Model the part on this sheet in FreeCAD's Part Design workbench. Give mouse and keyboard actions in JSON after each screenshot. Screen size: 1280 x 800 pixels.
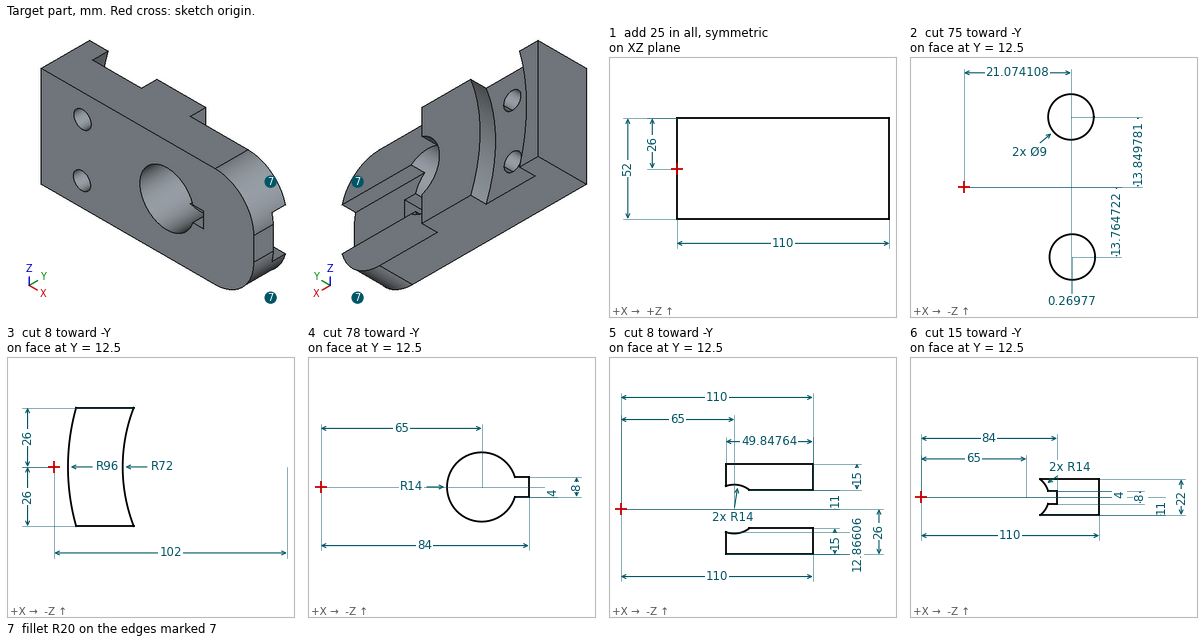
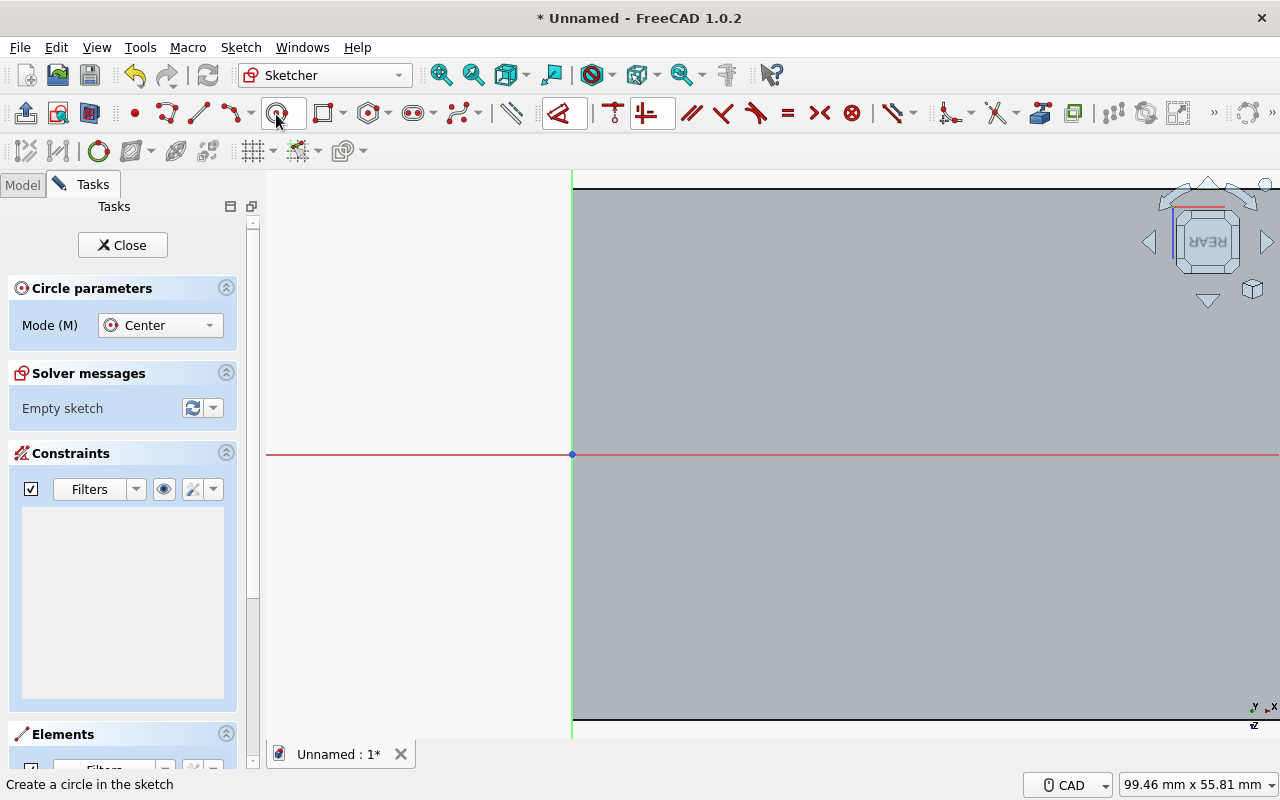
{"action": "left_click", "coordinate": [787, 313]}
{"action": "left_click", "coordinate": [820, 281]}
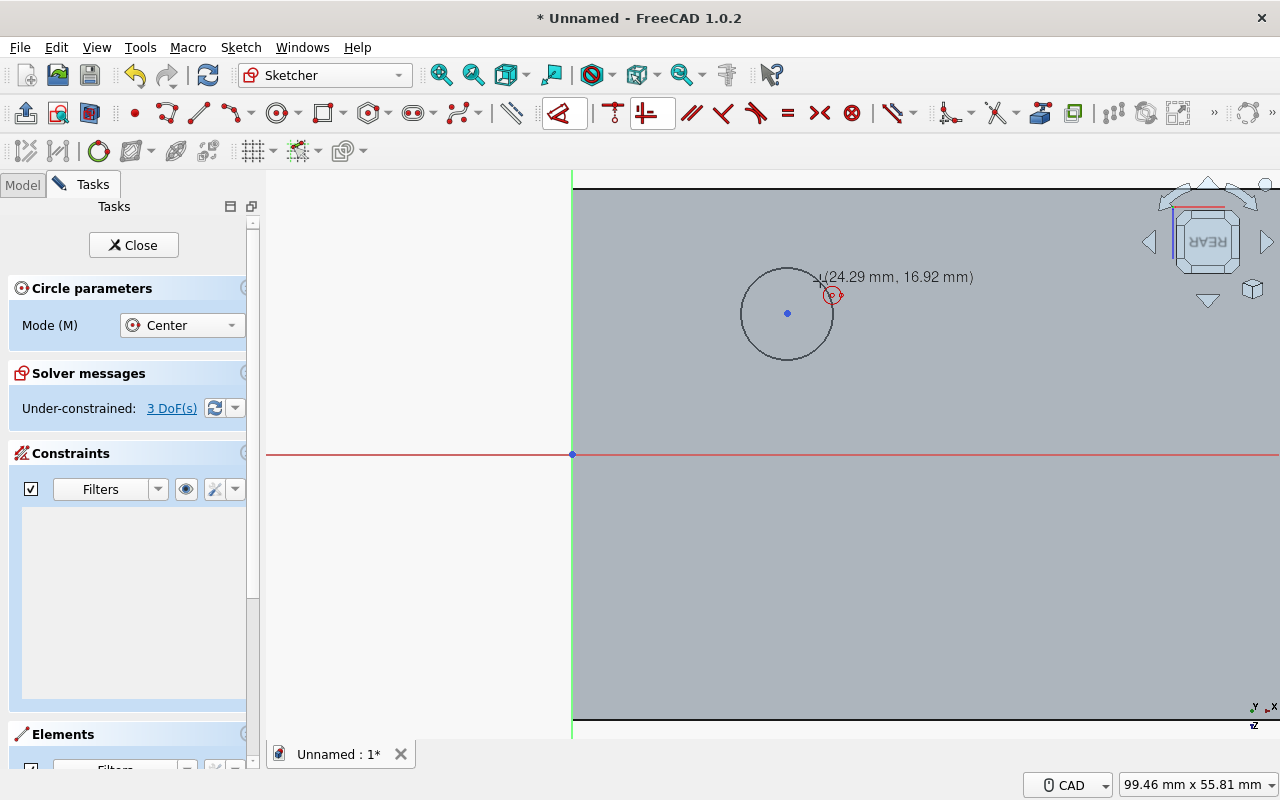
{"action": "left_click", "coordinate": [790, 595]}
{"action": "left_click", "coordinate": [822, 562]}
{"action": "key", "text": "Escape"}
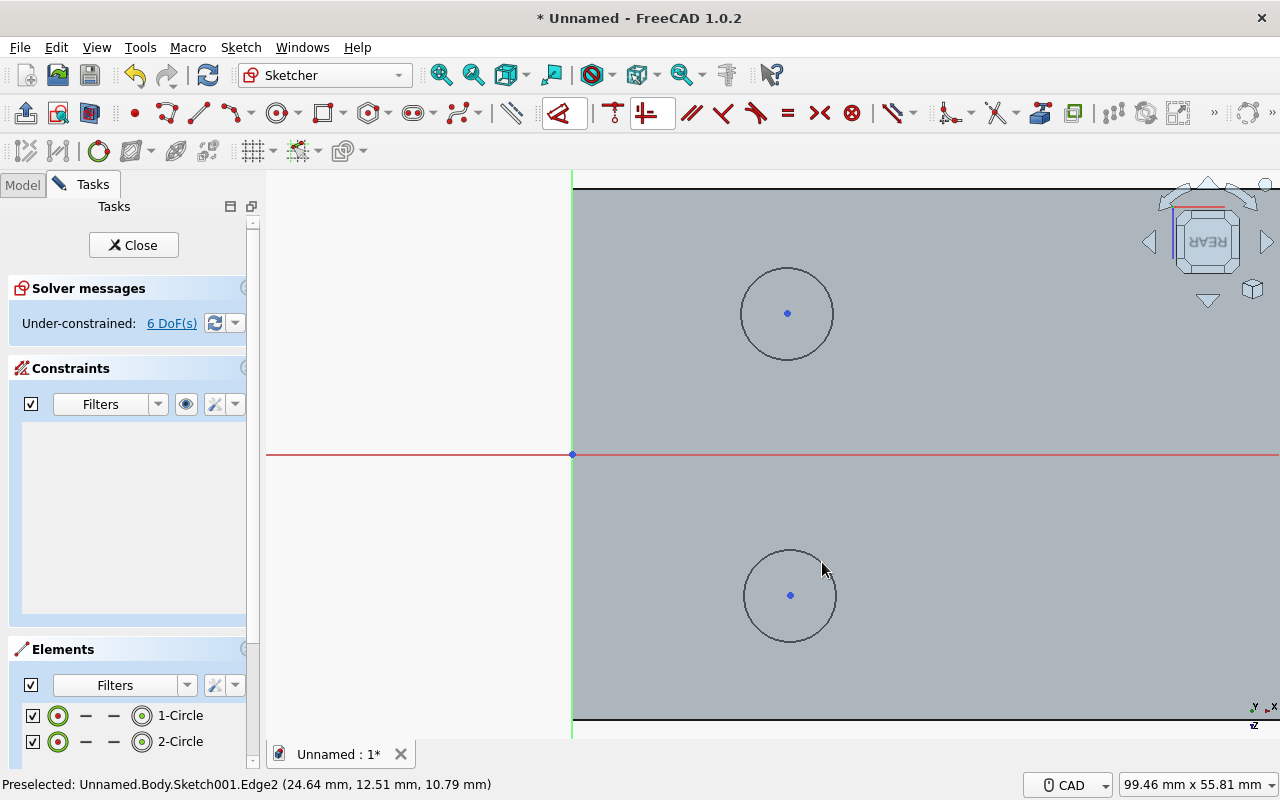
{"action": "left_click", "coordinate": [819, 281]}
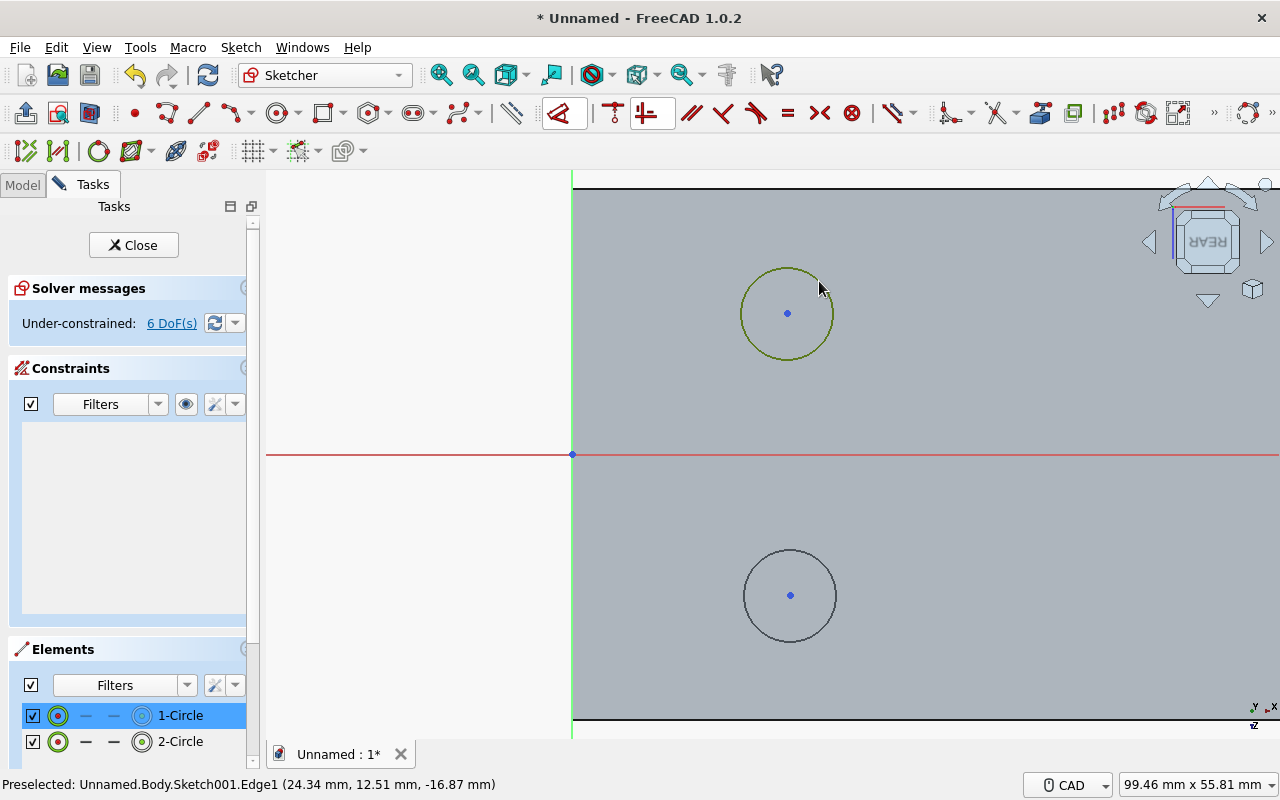
{"action": "left_click", "coordinate": [822, 563]}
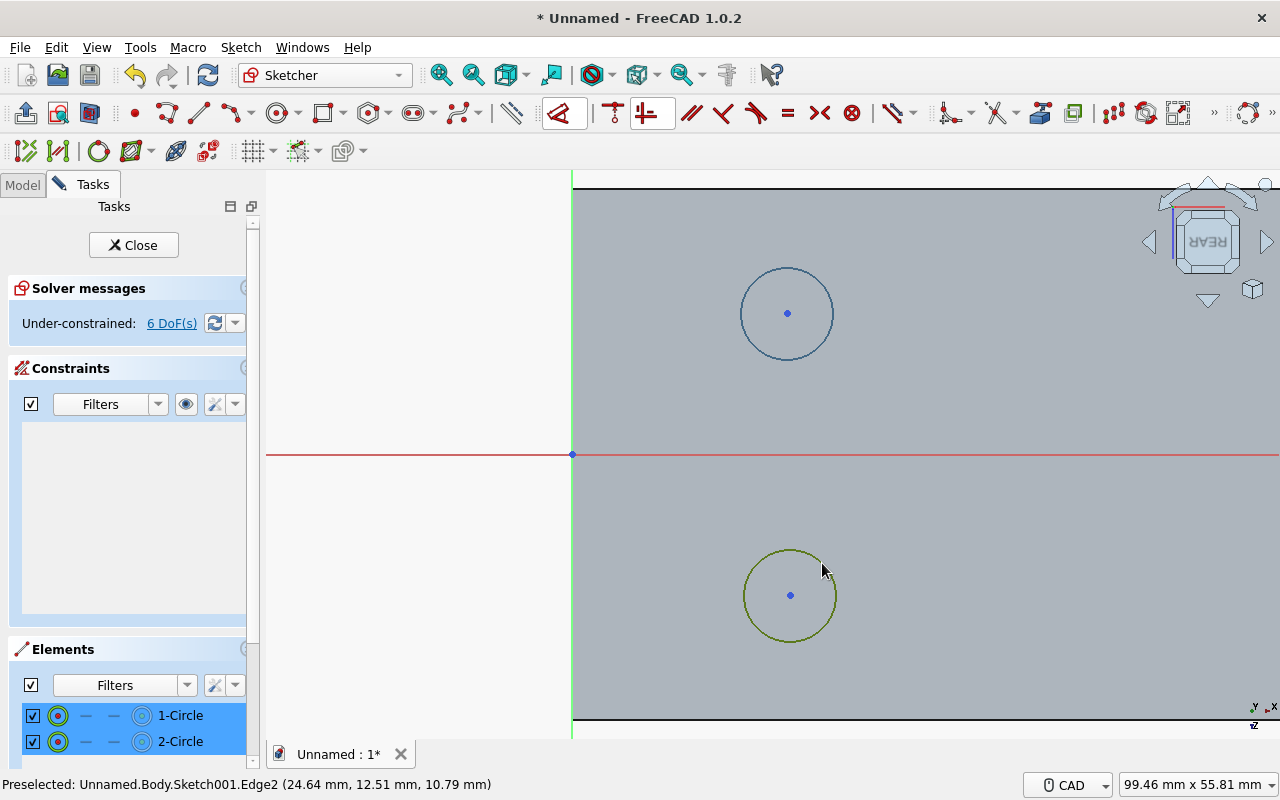
{"action": "left_click", "coordinate": [788, 114]}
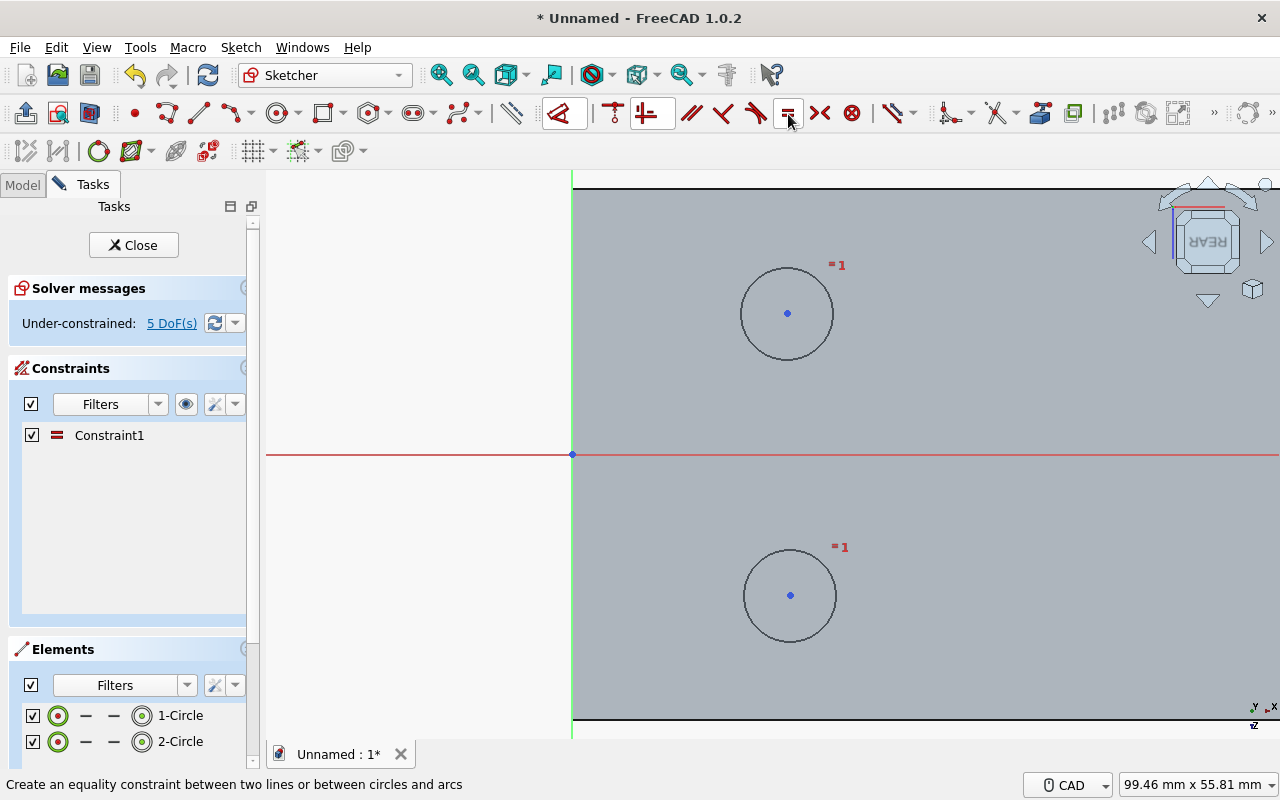
{"action": "left_click", "coordinate": [819, 281]}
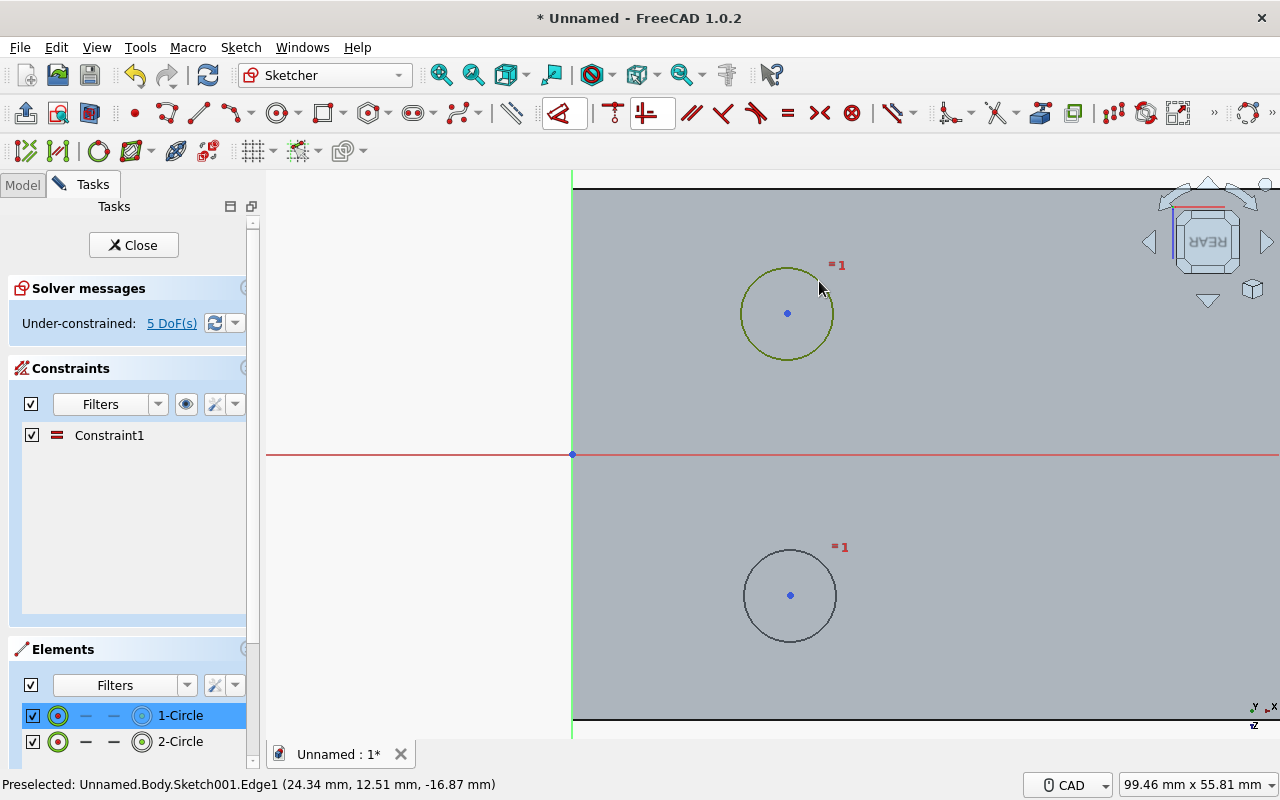
{"action": "left_click", "coordinate": [582, 114]}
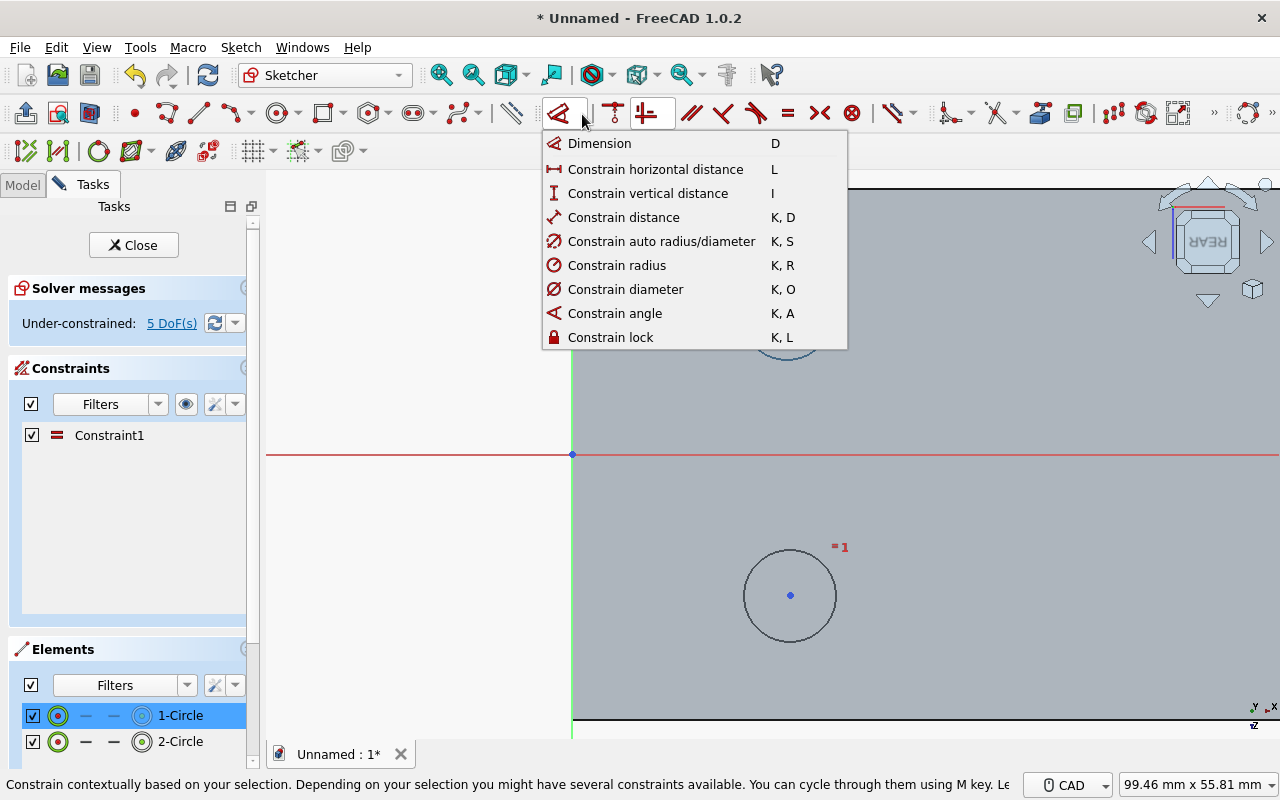
{"action": "left_click", "coordinate": [695, 289]}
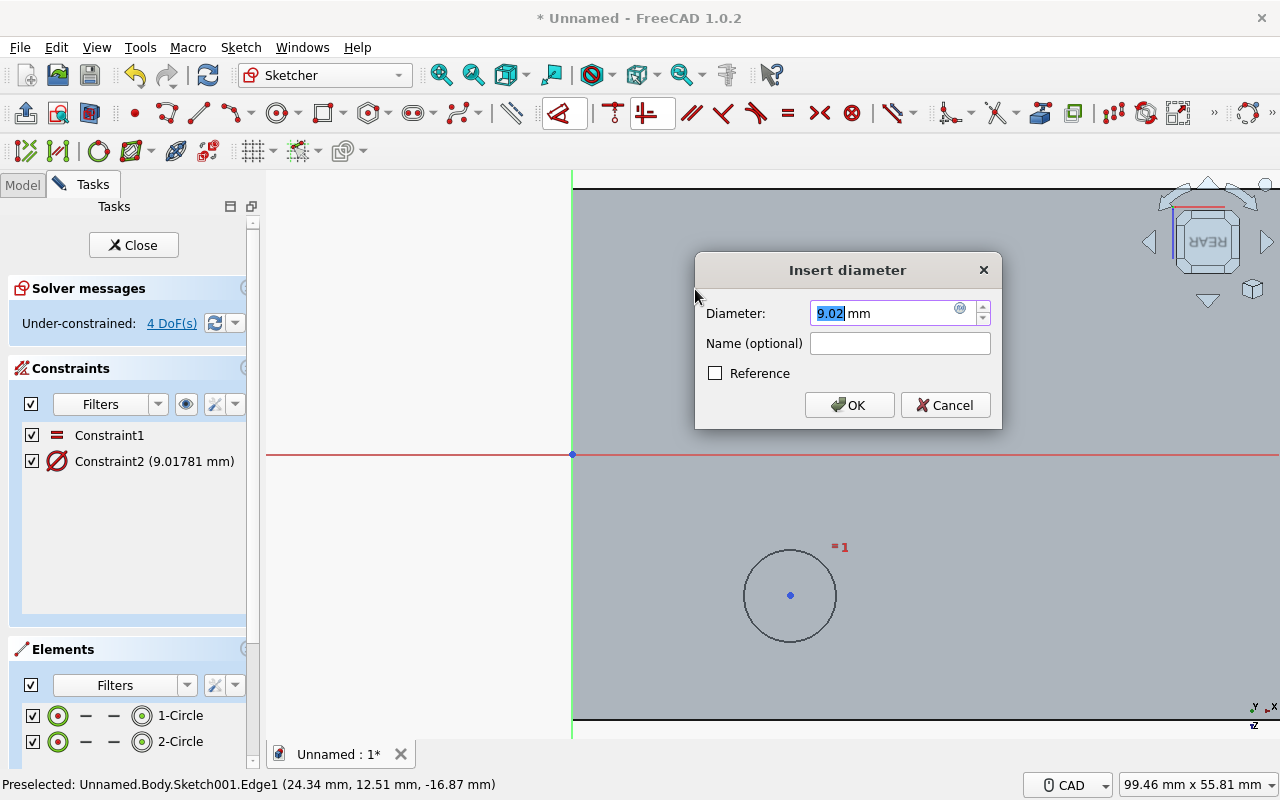
{"action": "type", "text": "9"}
{"action": "key", "text": "Return"}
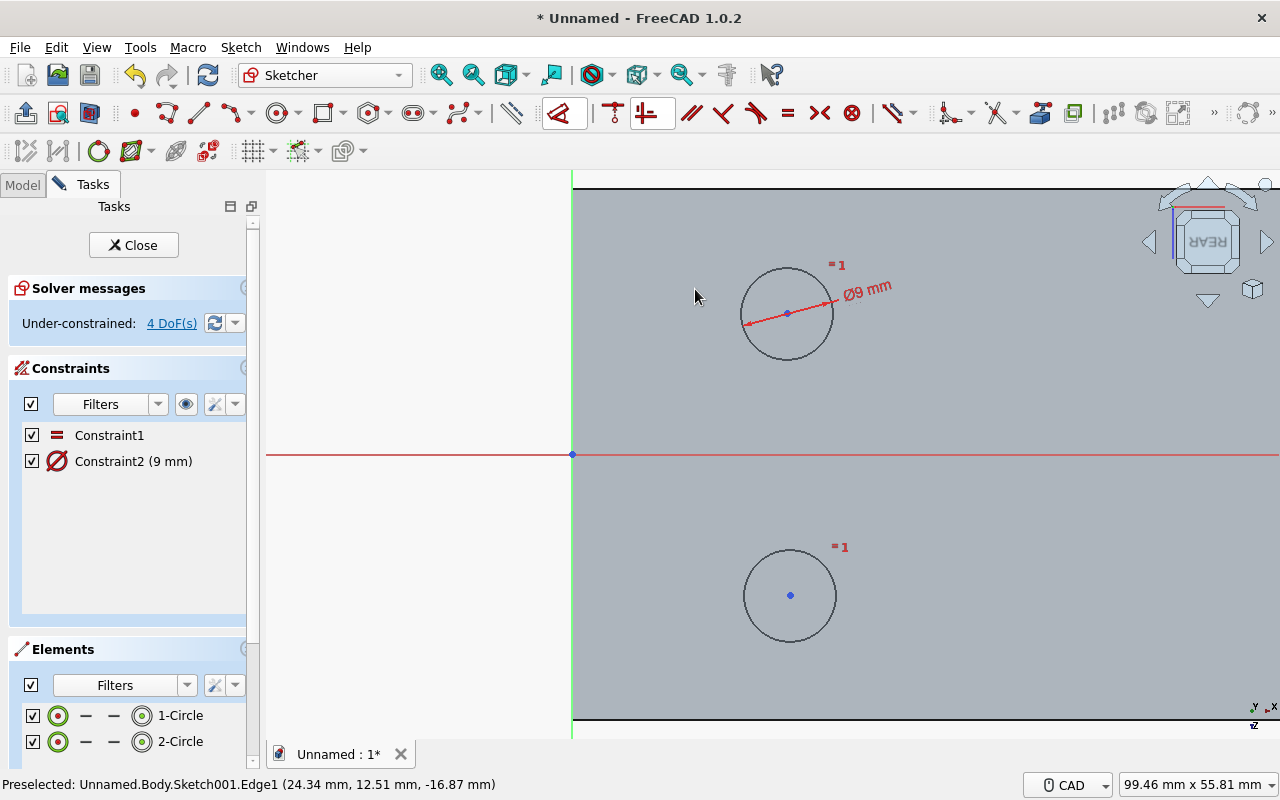
{"action": "scroll", "coordinate": [787, 314], "scroll_direction": "up", "scroll_amount": 14}